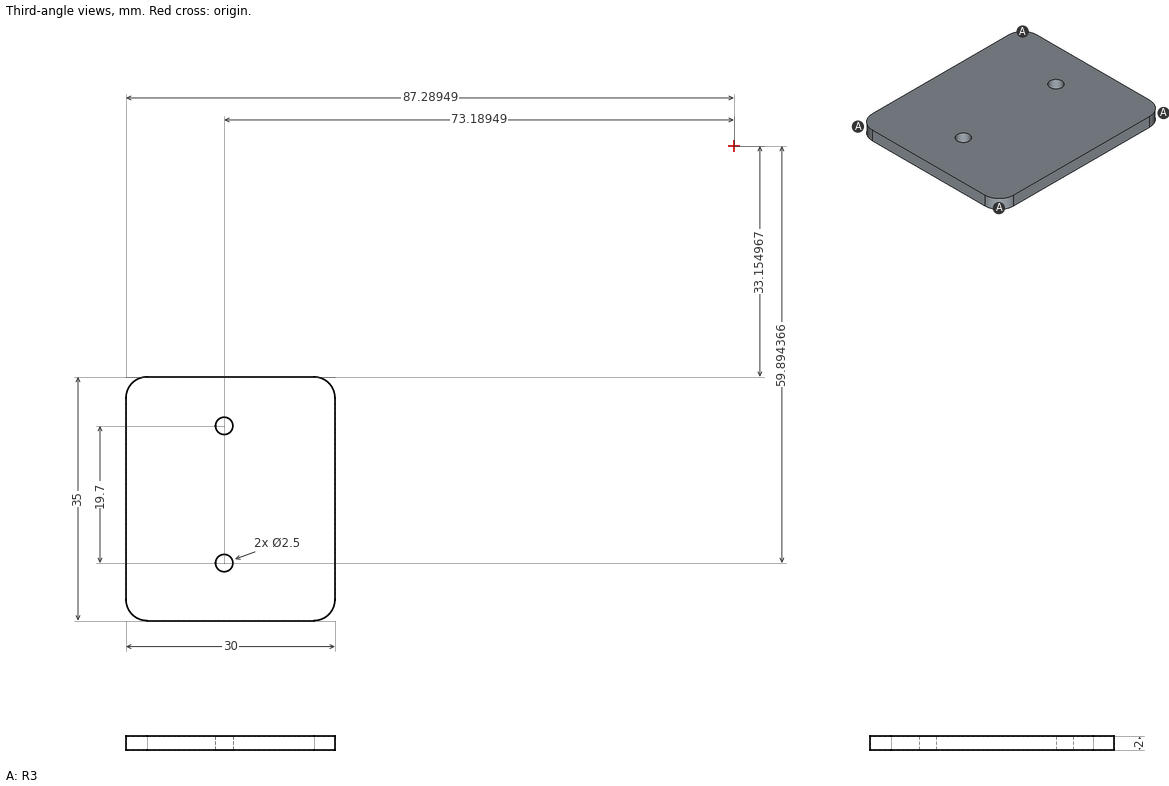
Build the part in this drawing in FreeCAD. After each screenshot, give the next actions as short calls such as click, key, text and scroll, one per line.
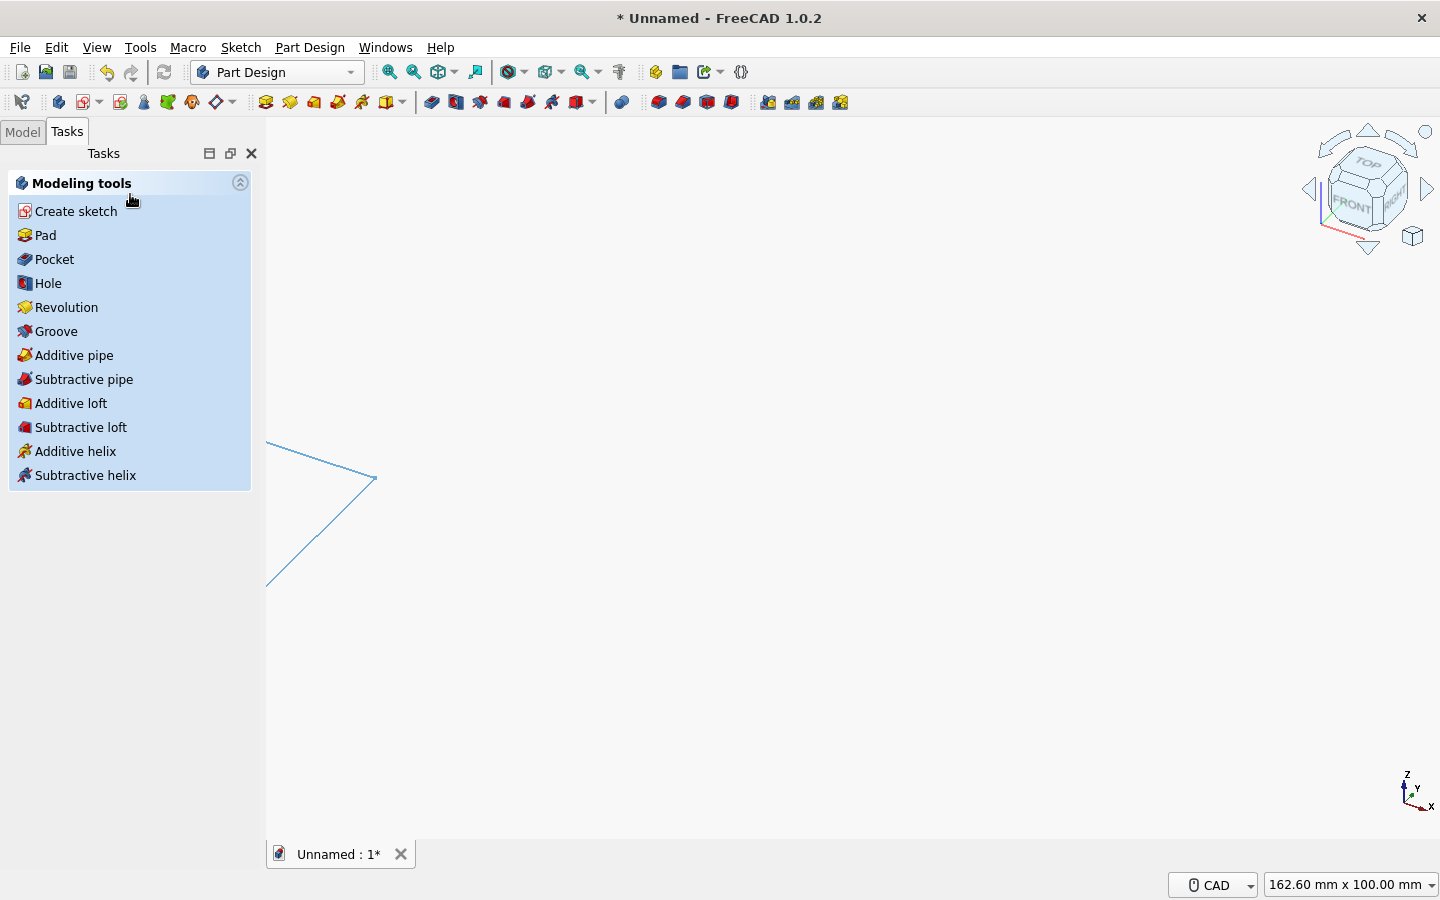
click(266, 102)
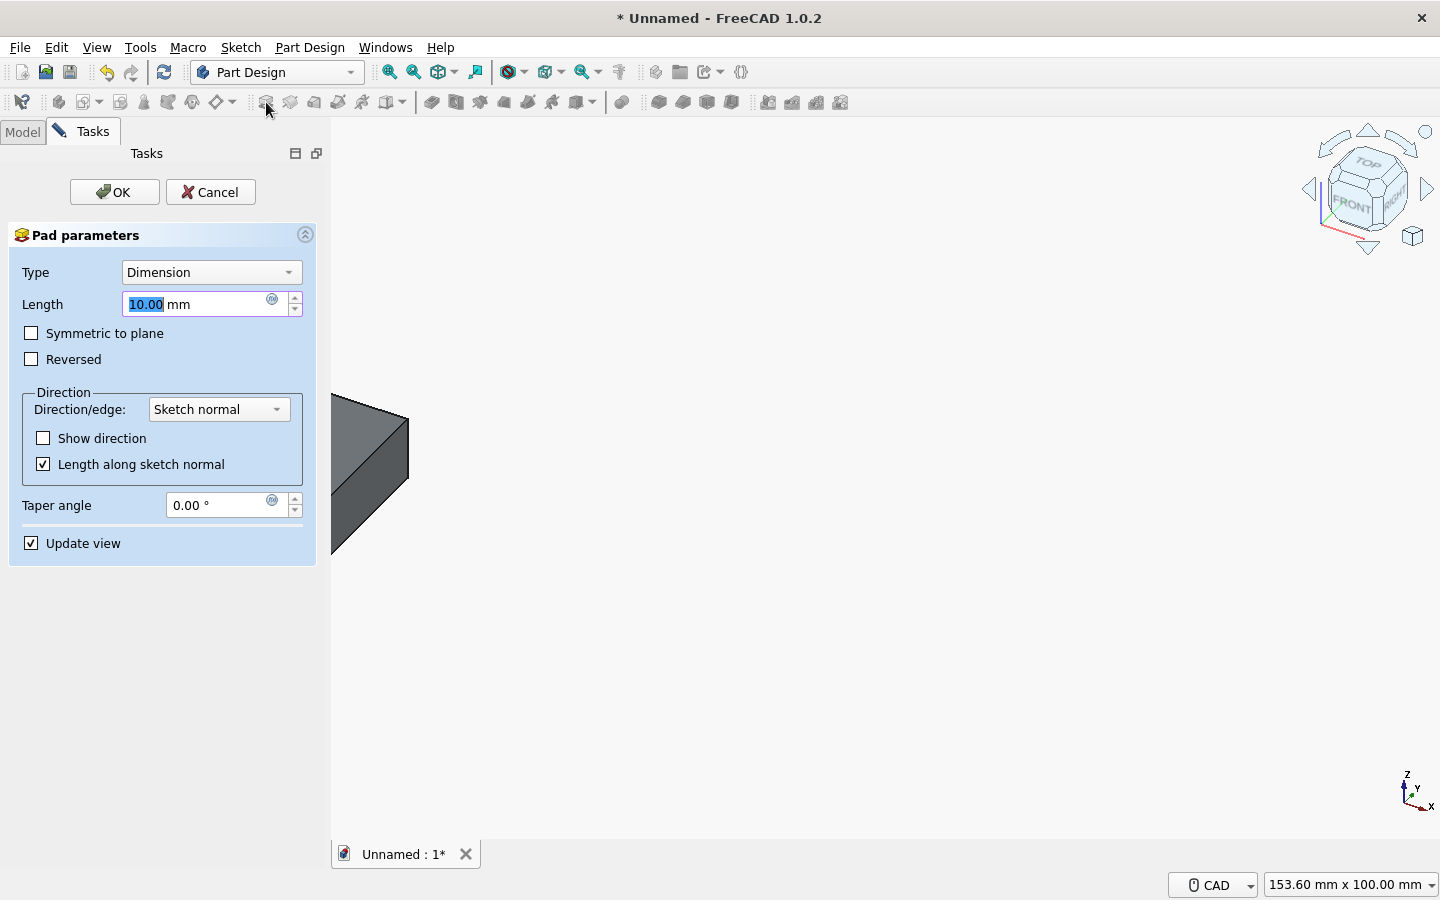
text(2)
key(Tab)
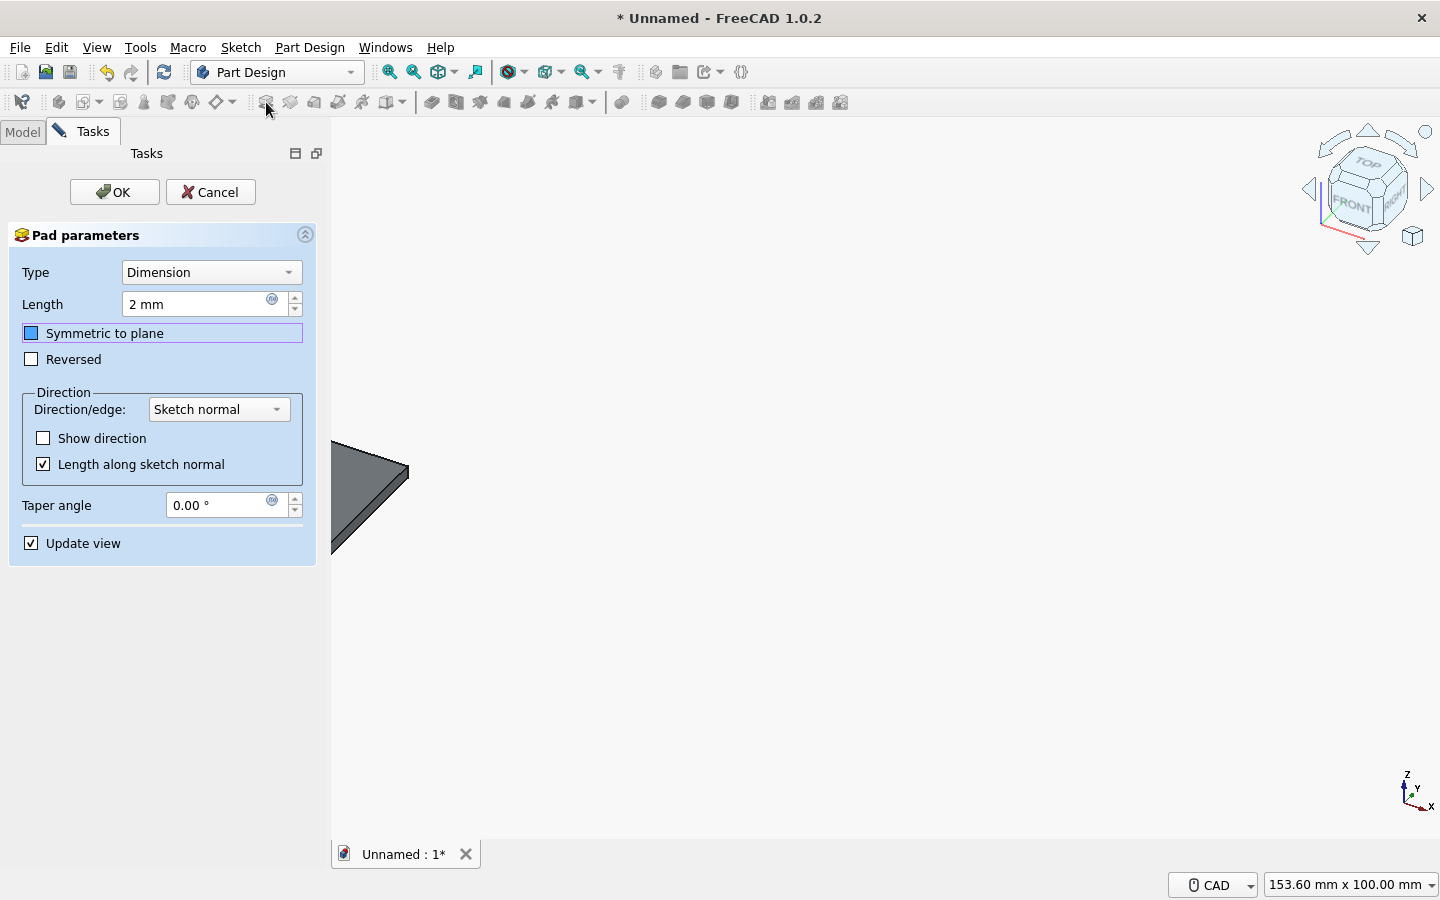
click(115, 192)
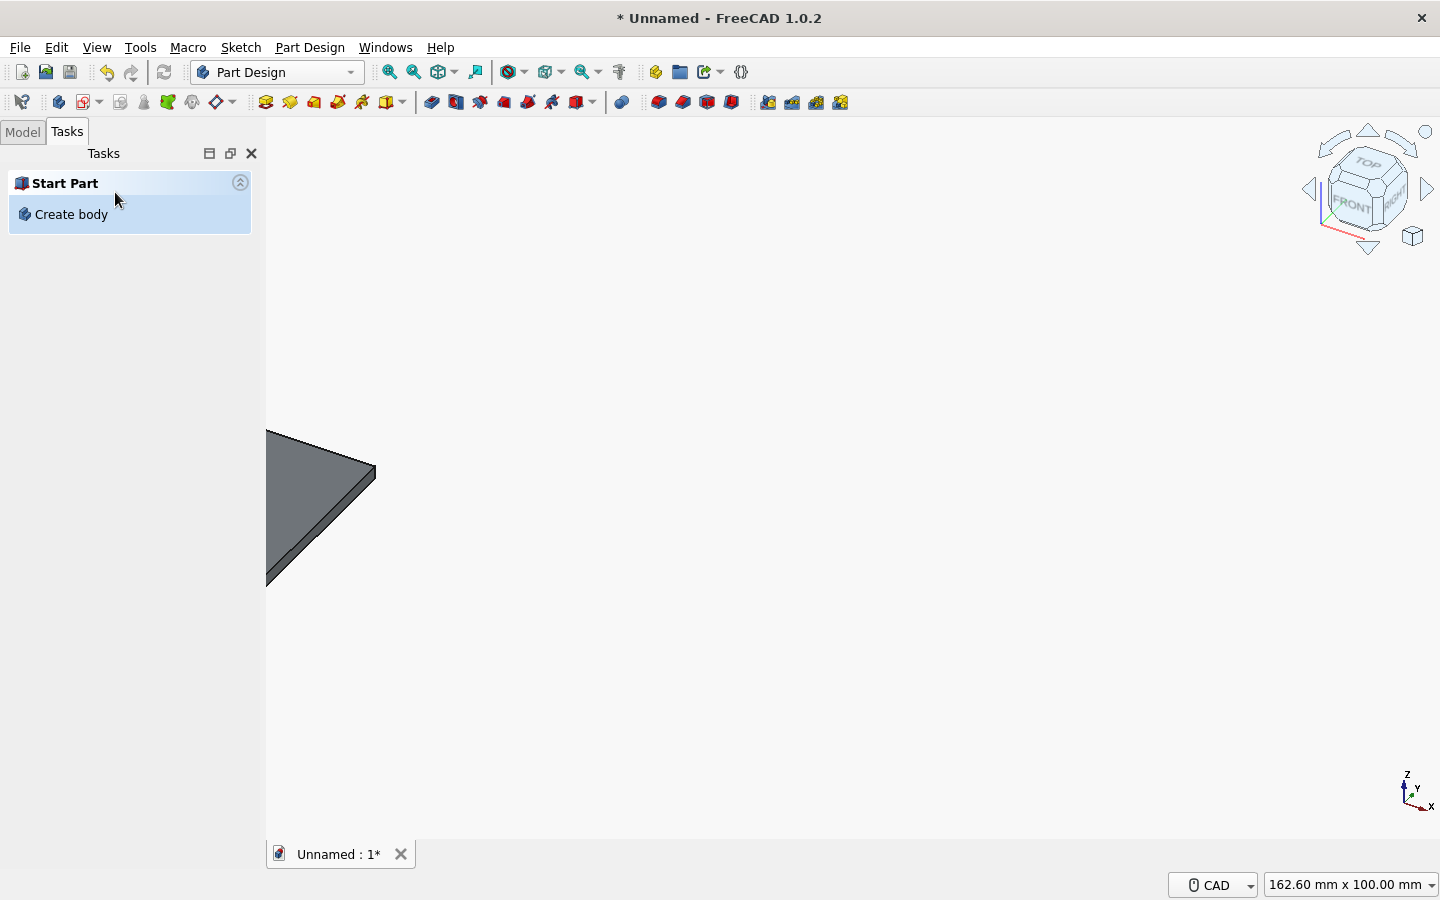
click(390, 72)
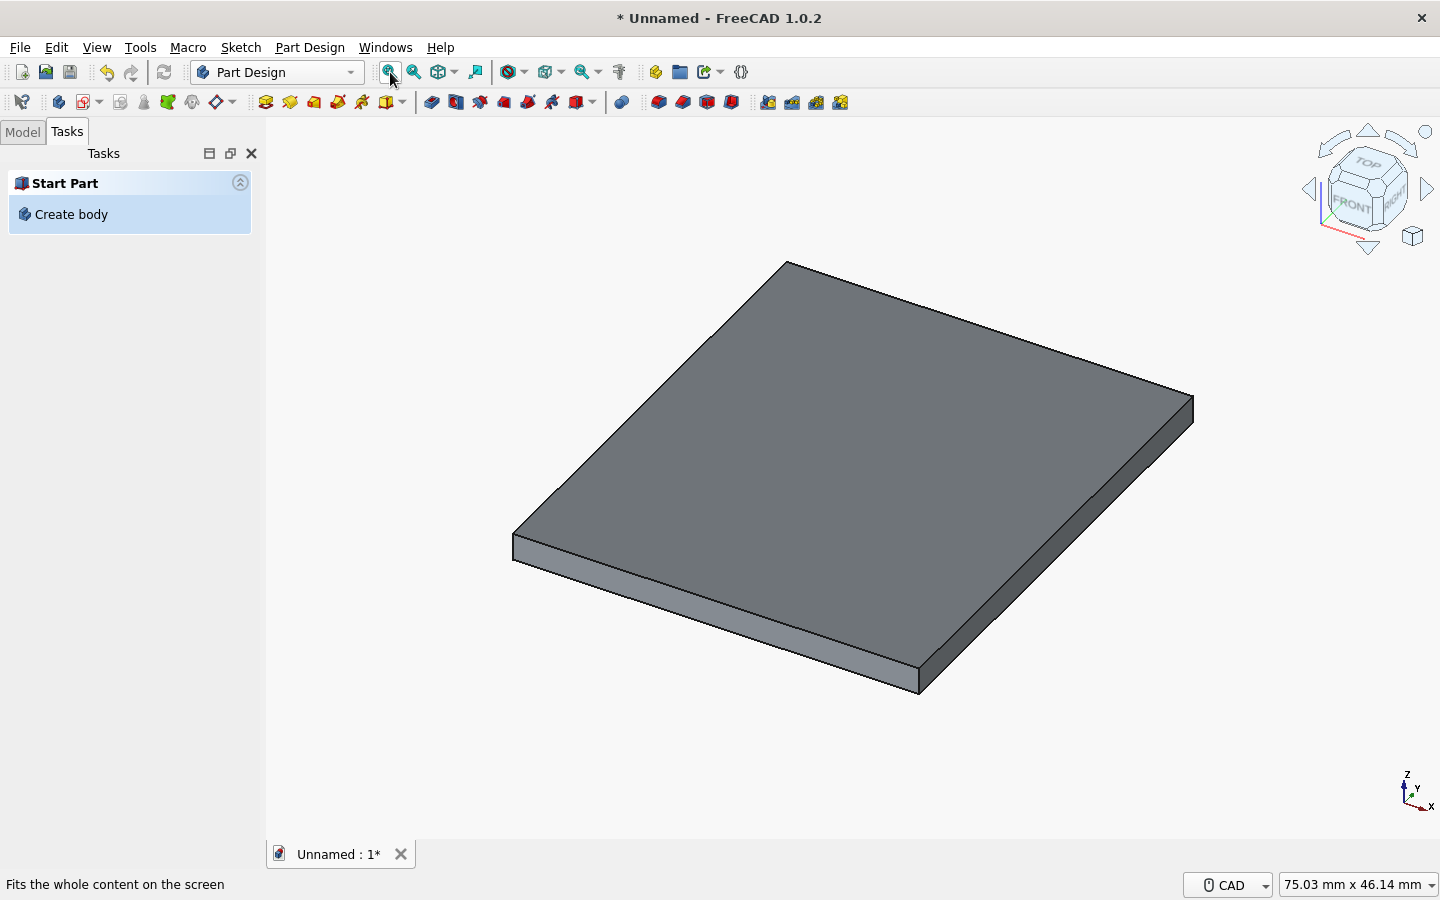
click(919, 680)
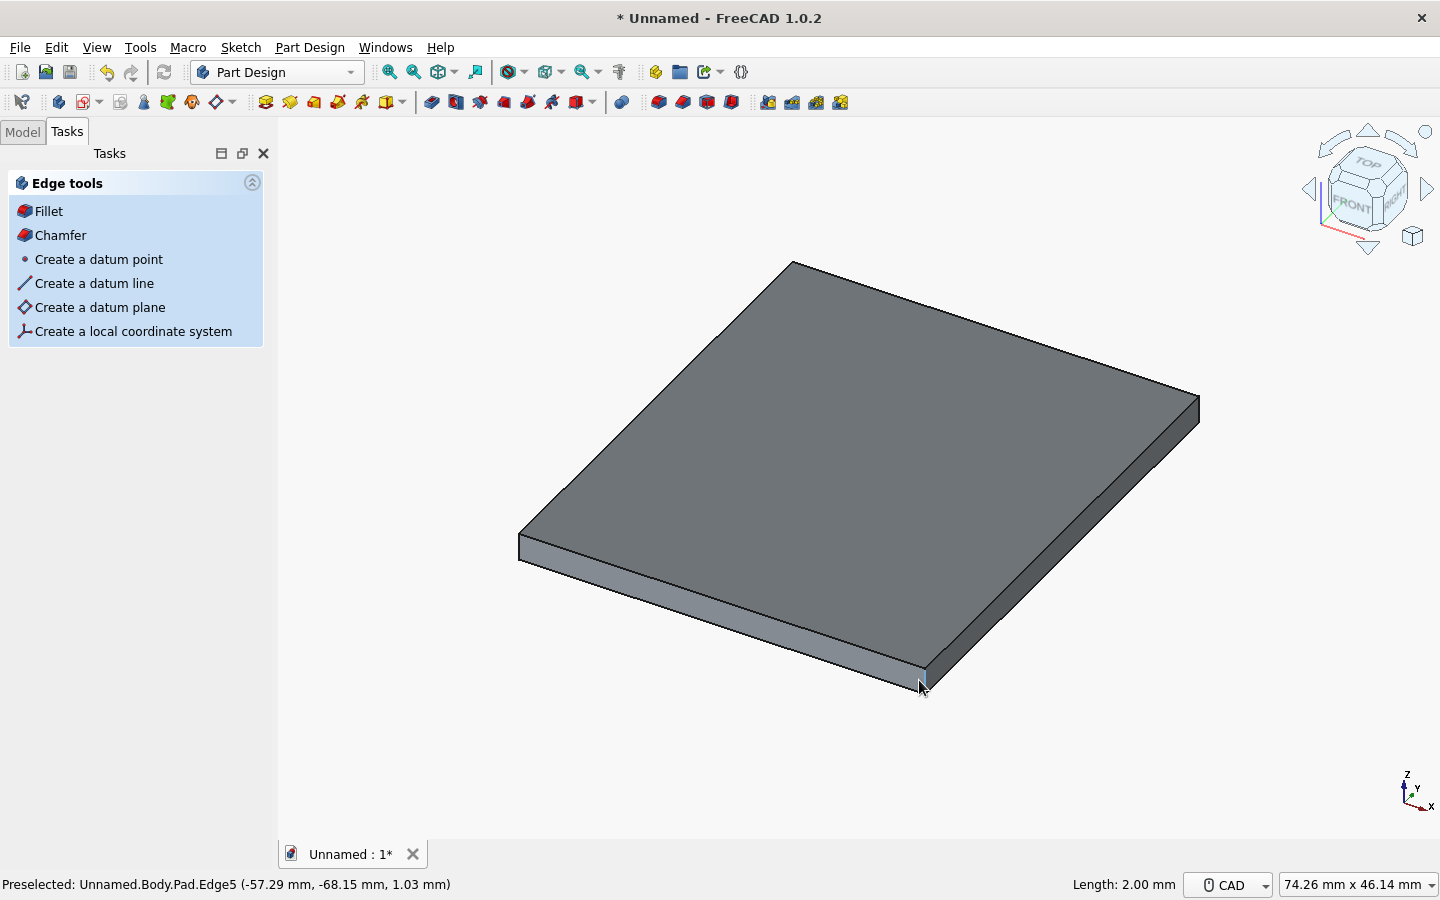
key(0)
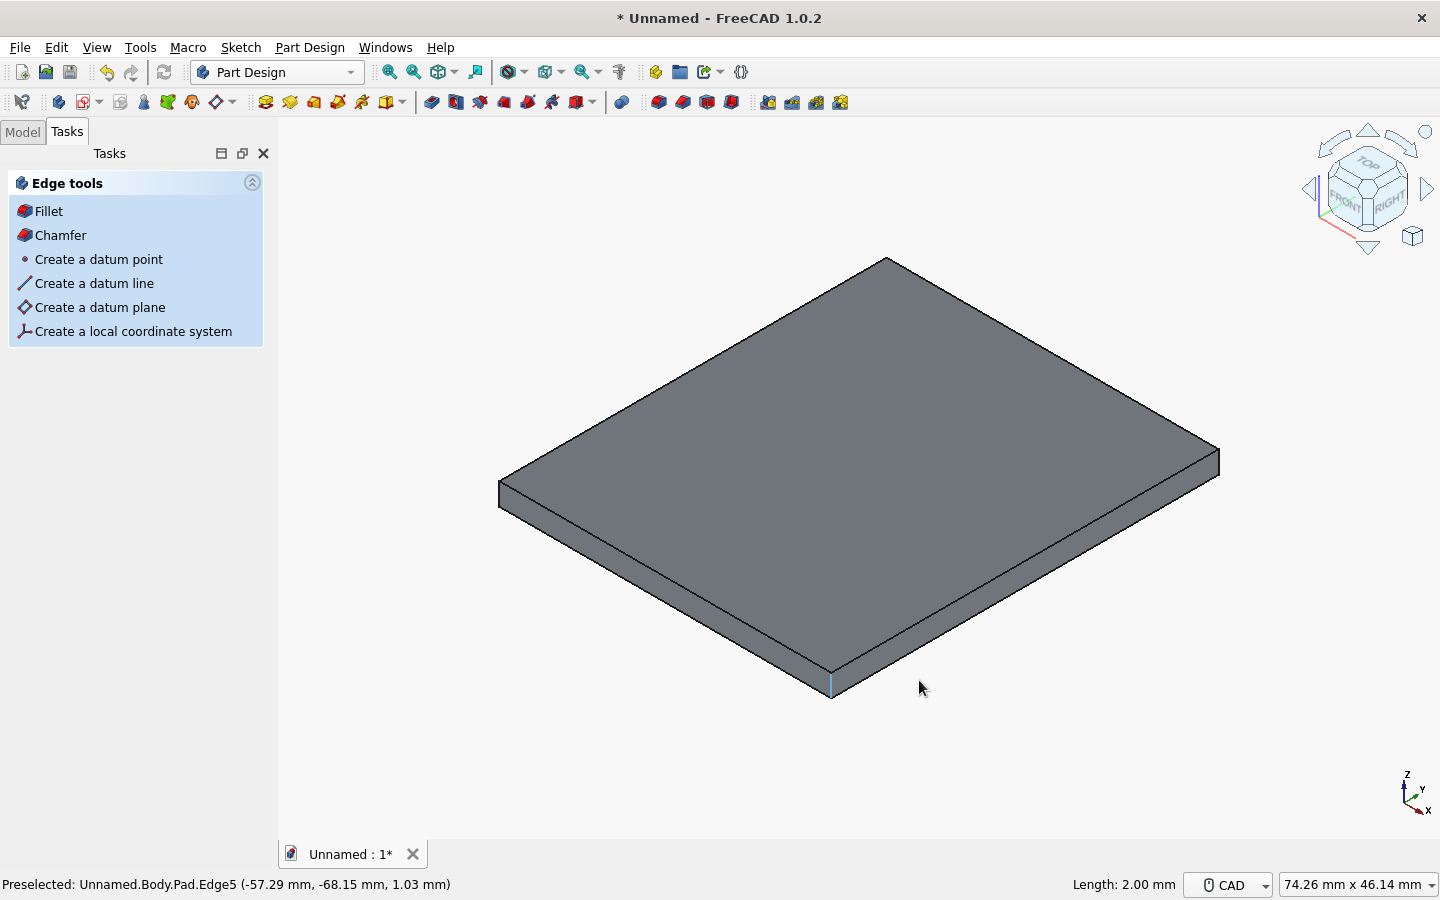
key(2)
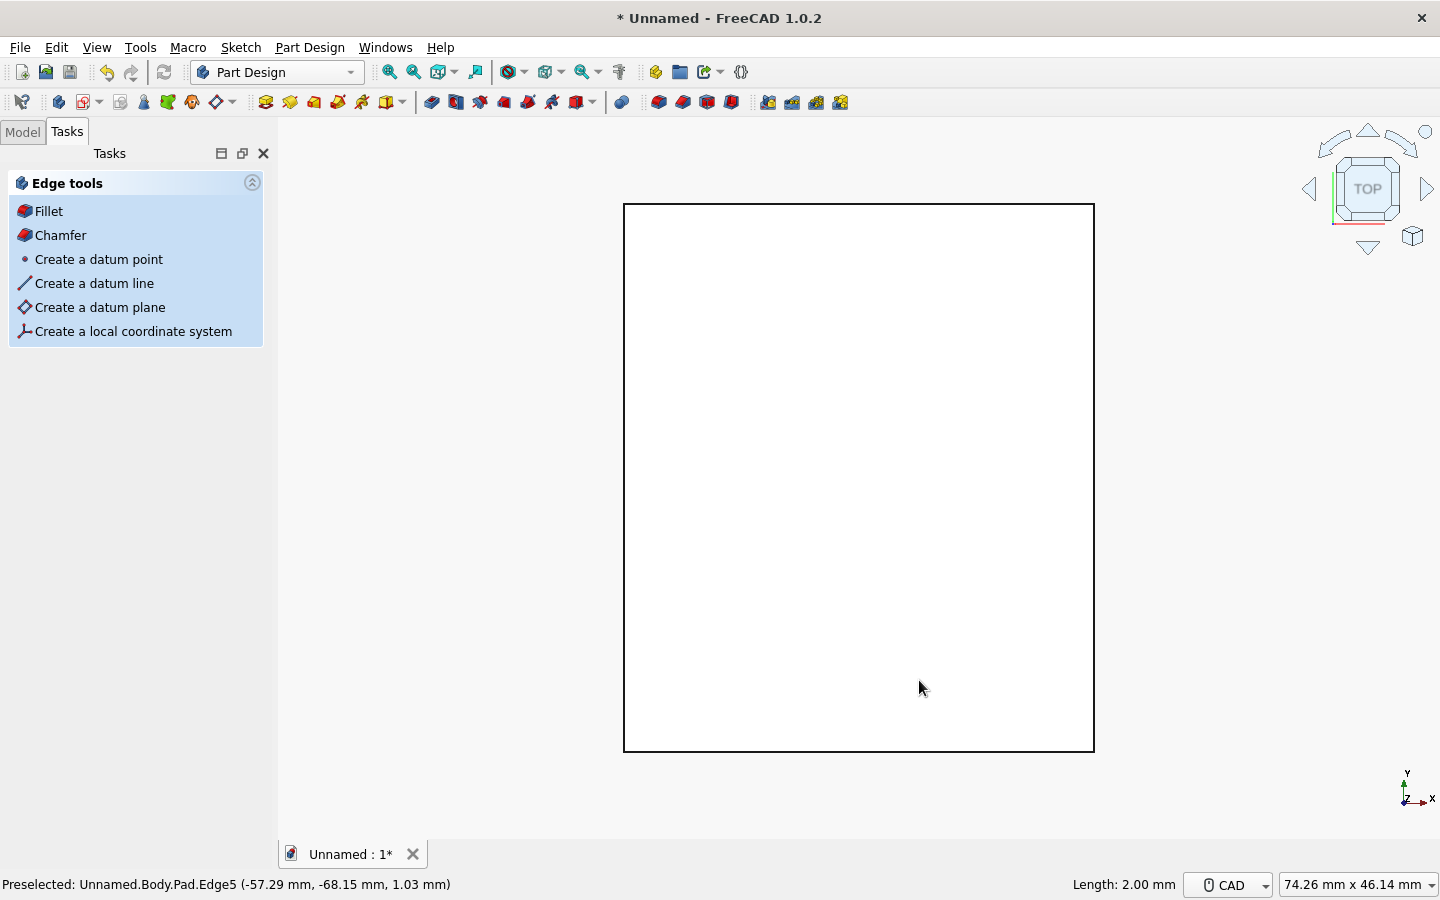
key(1)